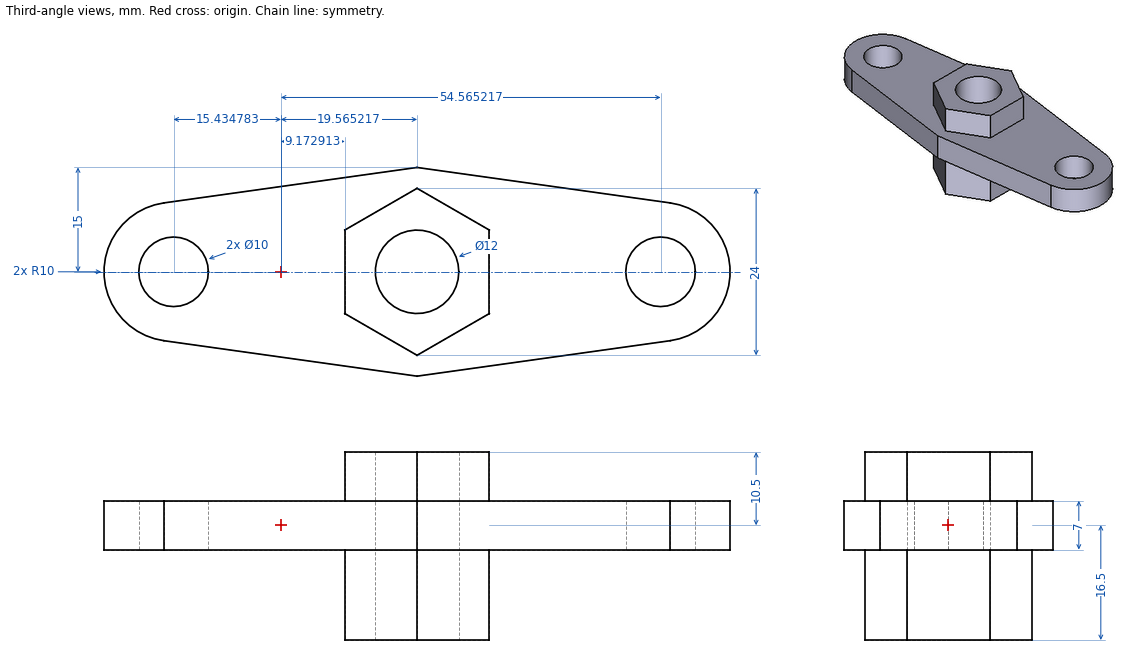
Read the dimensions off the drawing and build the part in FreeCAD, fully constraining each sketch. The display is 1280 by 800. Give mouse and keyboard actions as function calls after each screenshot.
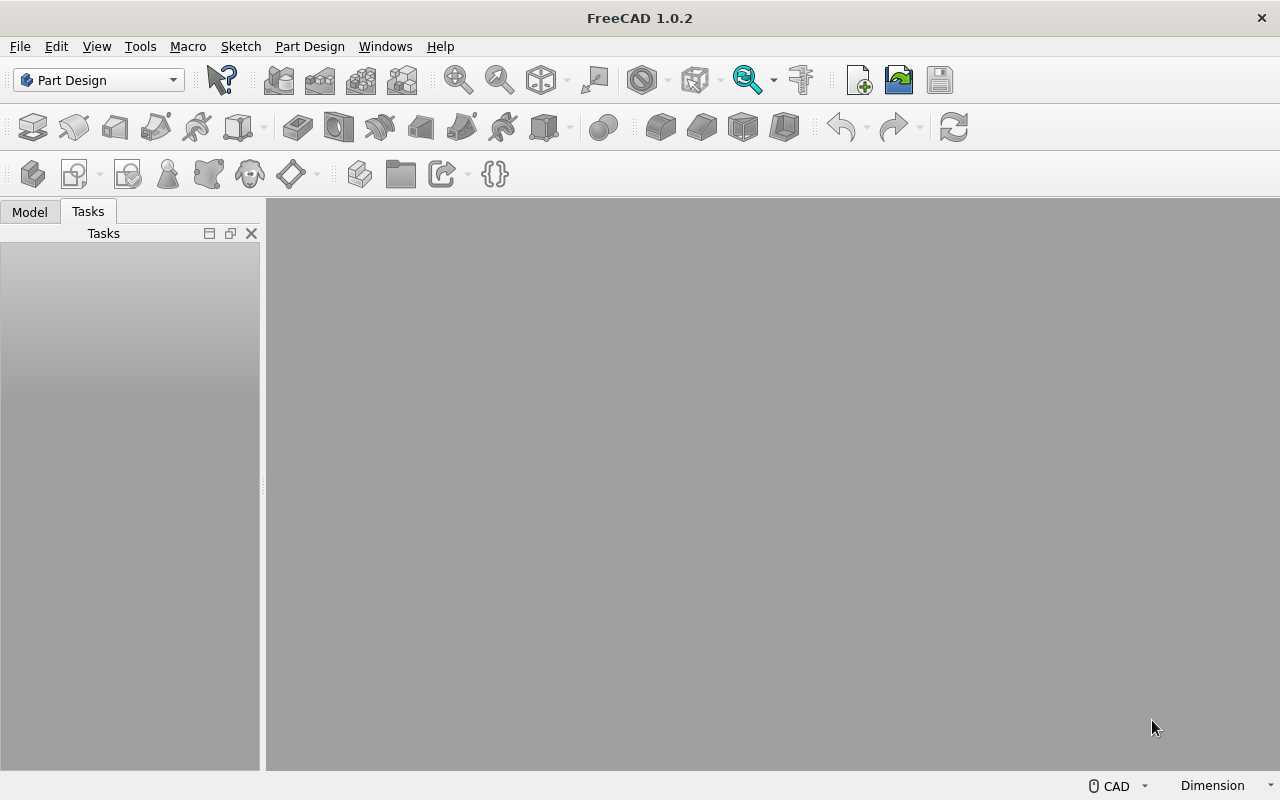
click(858, 80)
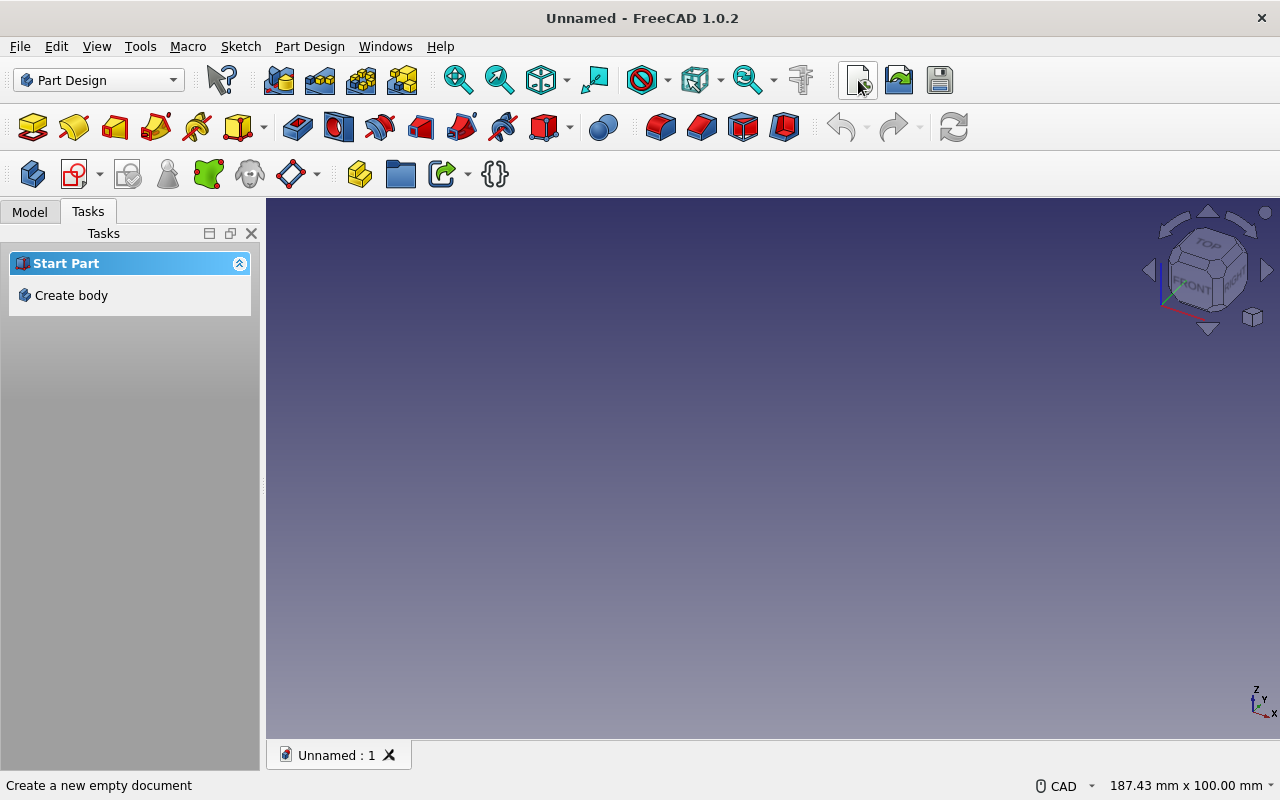
click(74, 174)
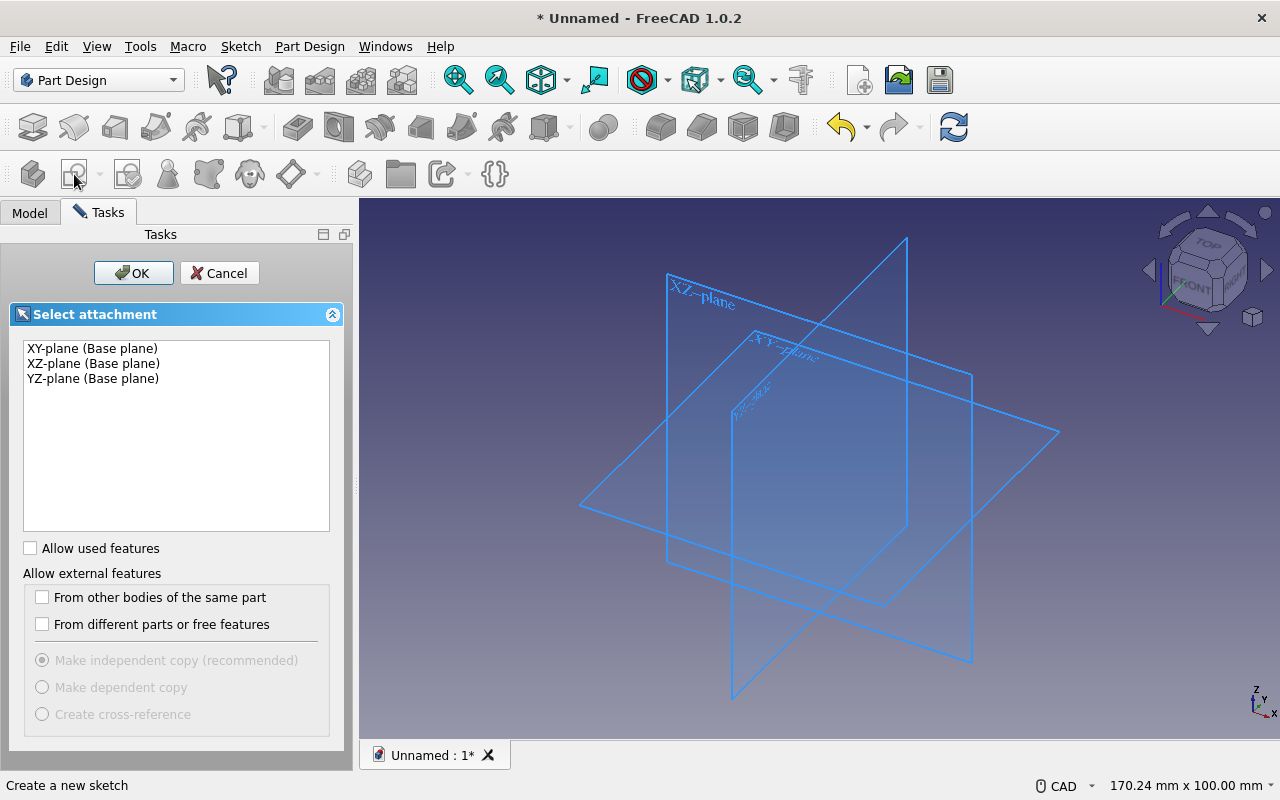
click(84, 348)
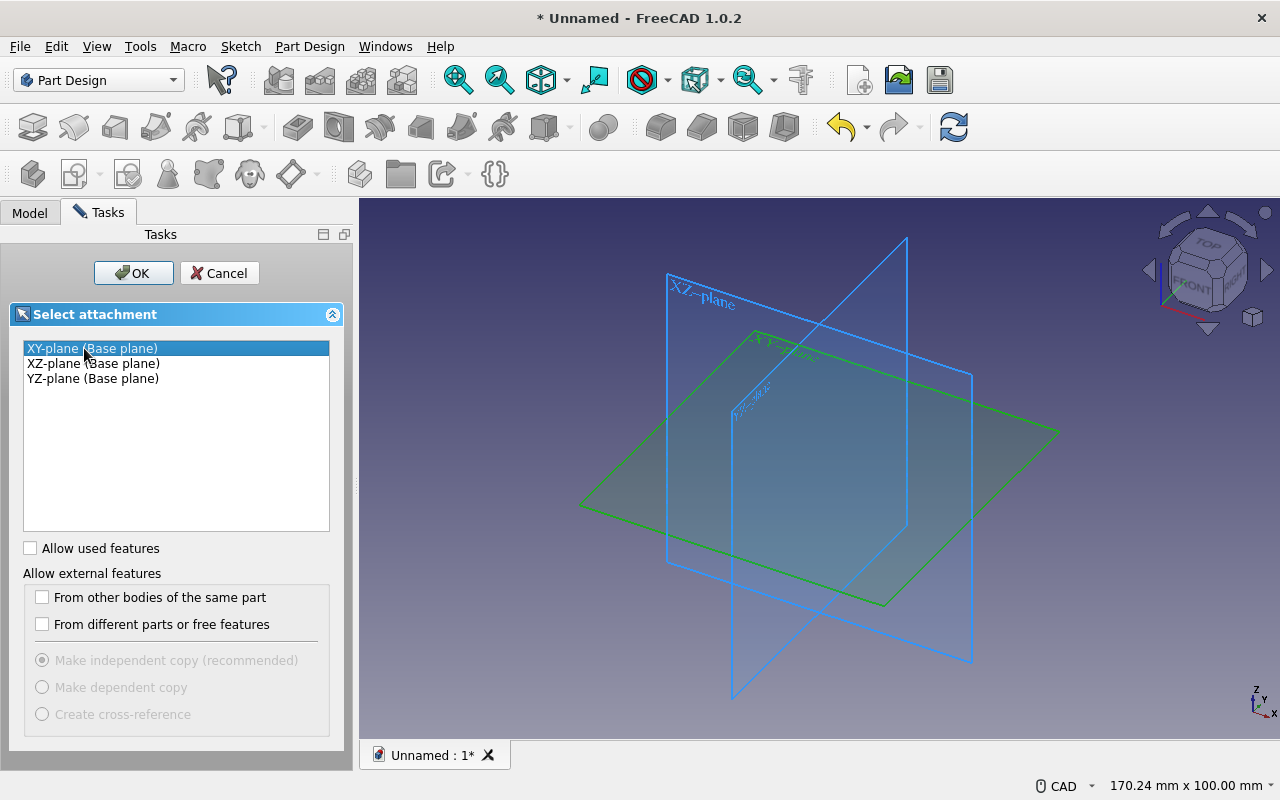
click(134, 273)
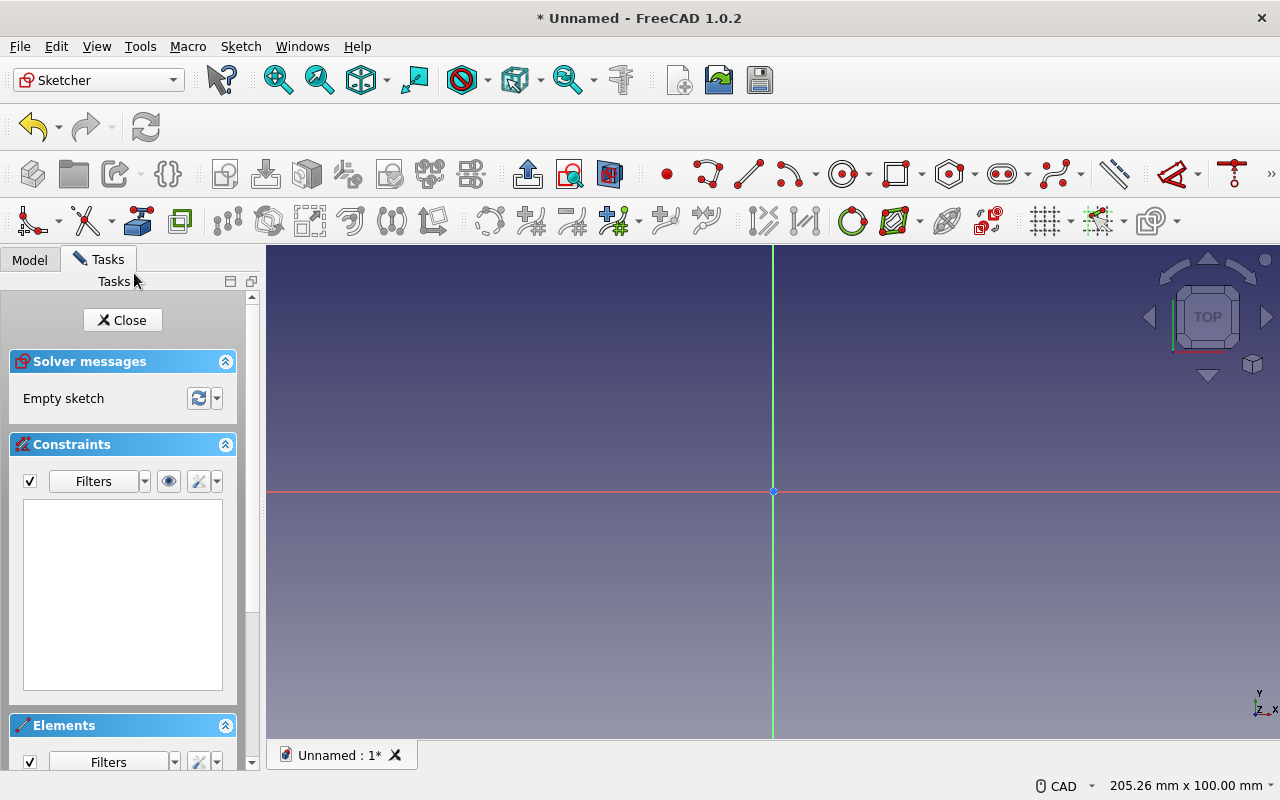
scroll(1115, 492, up, 1)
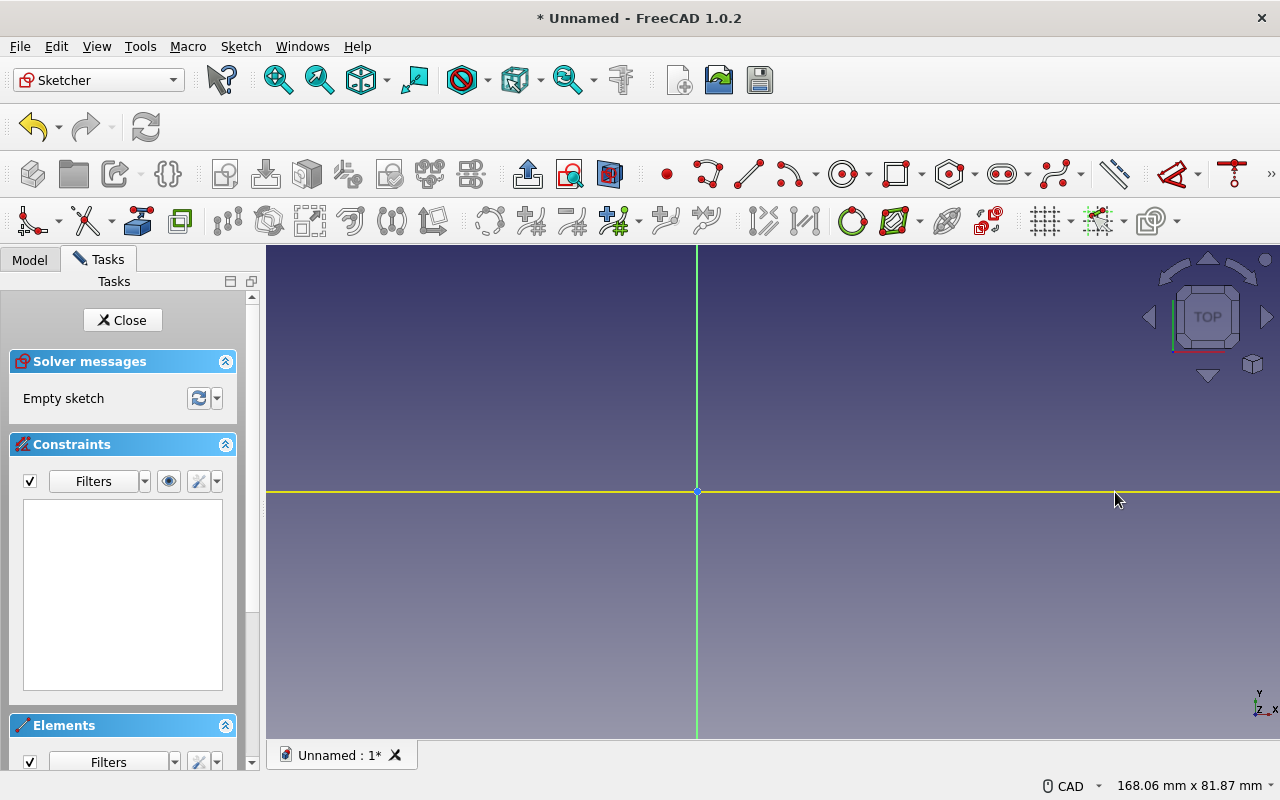
click(708, 174)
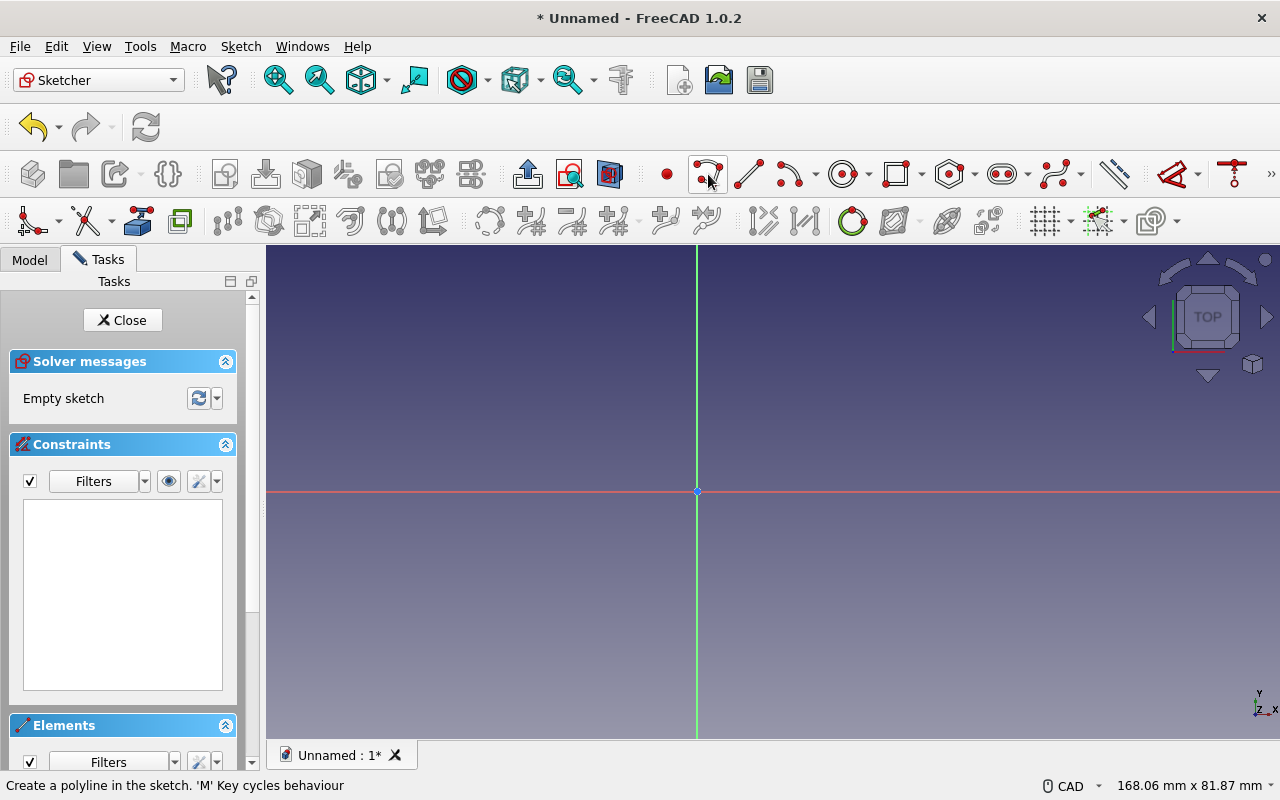
click(1035, 432)
click(815, 401)
click(596, 432)
right_click(596, 432)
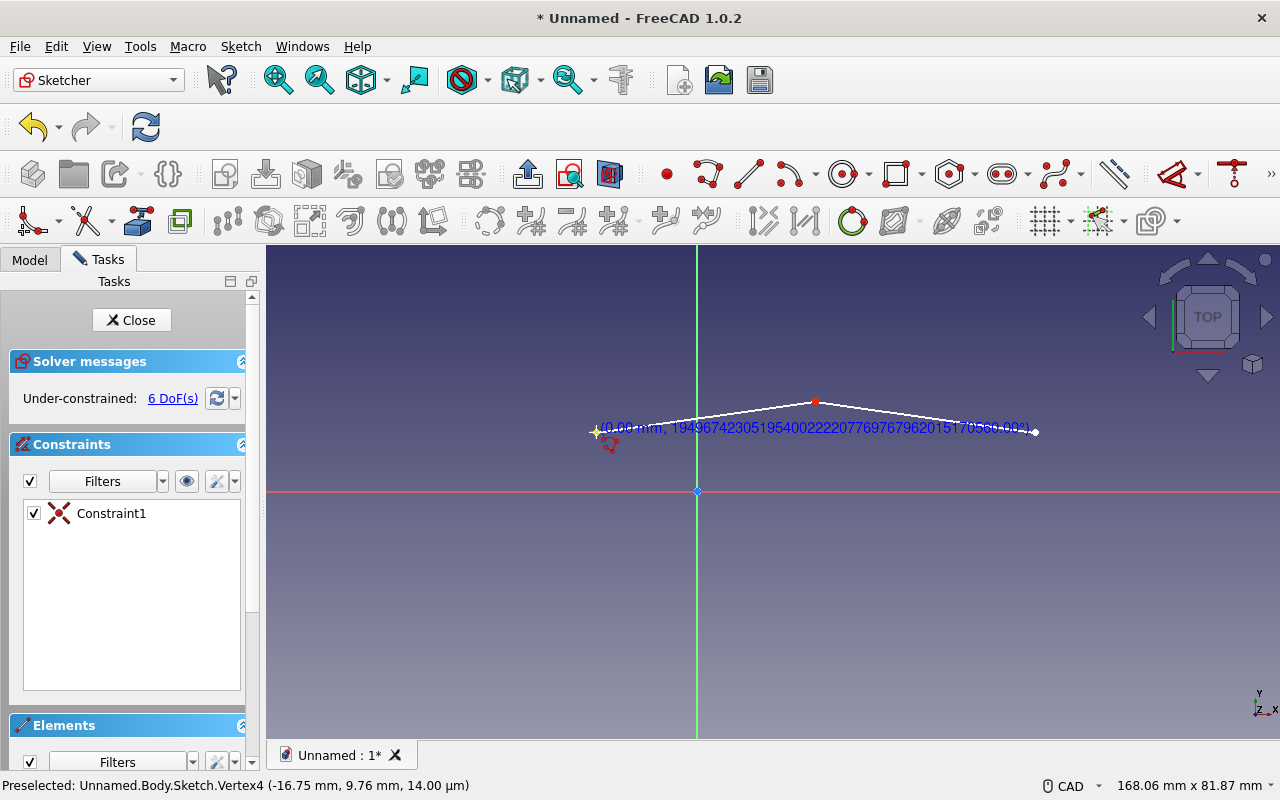
click(596, 552)
click(815, 582)
click(1035, 552)
right_click(1035, 552)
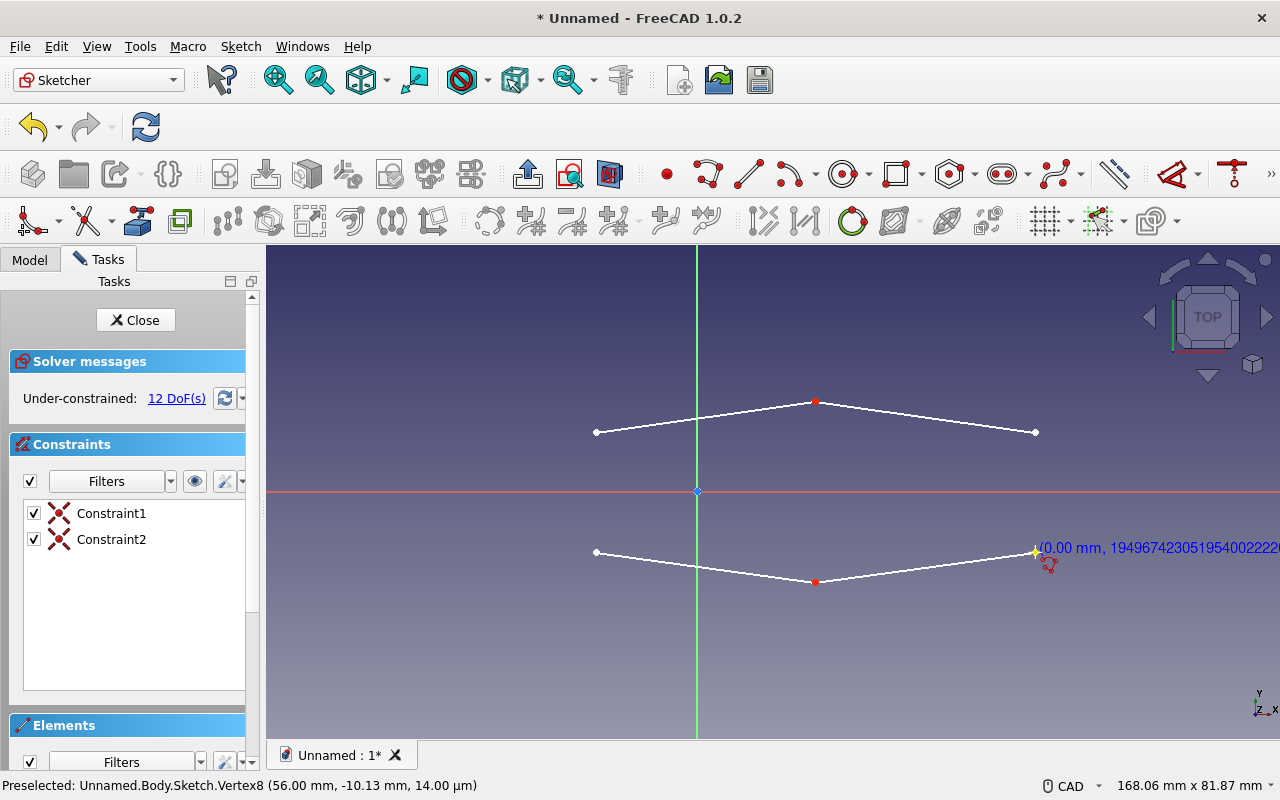
key(g)
key(3)
key(a)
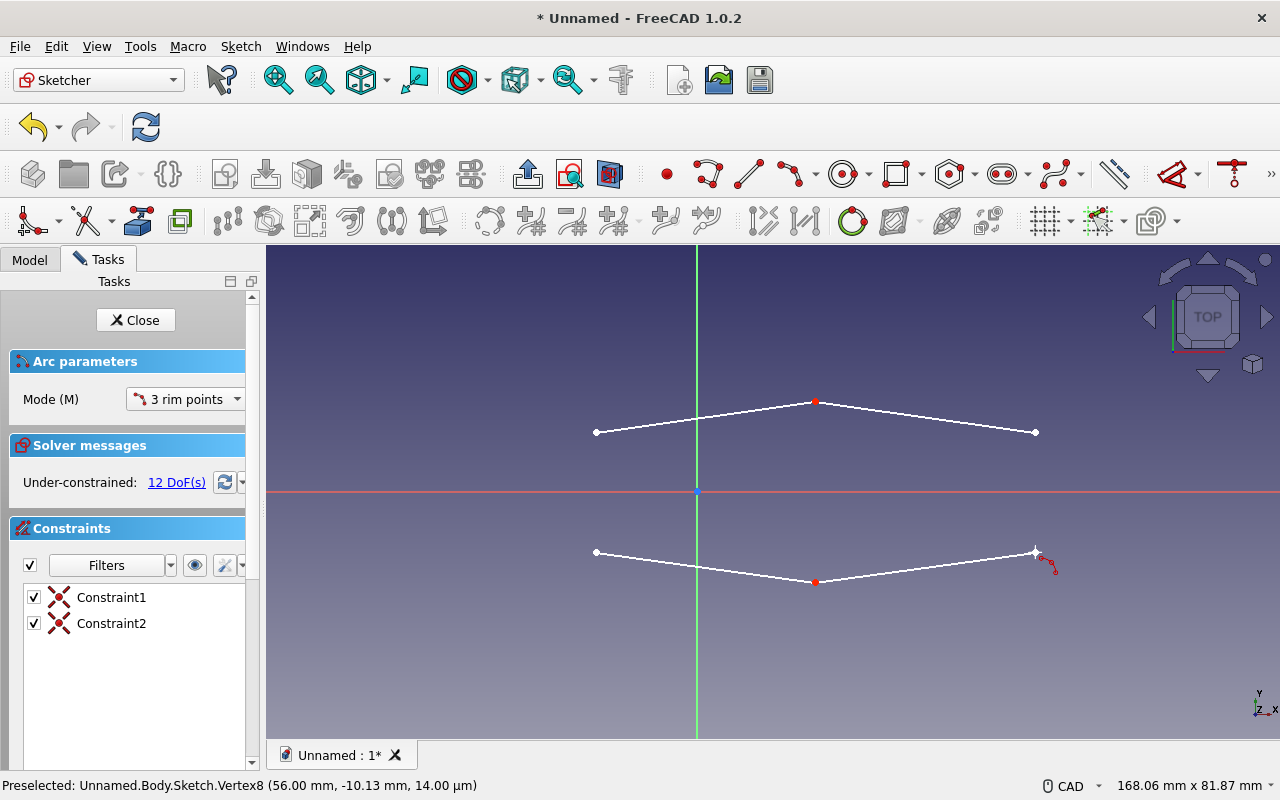
click(596, 433)
click(596, 553)
click(546, 475)